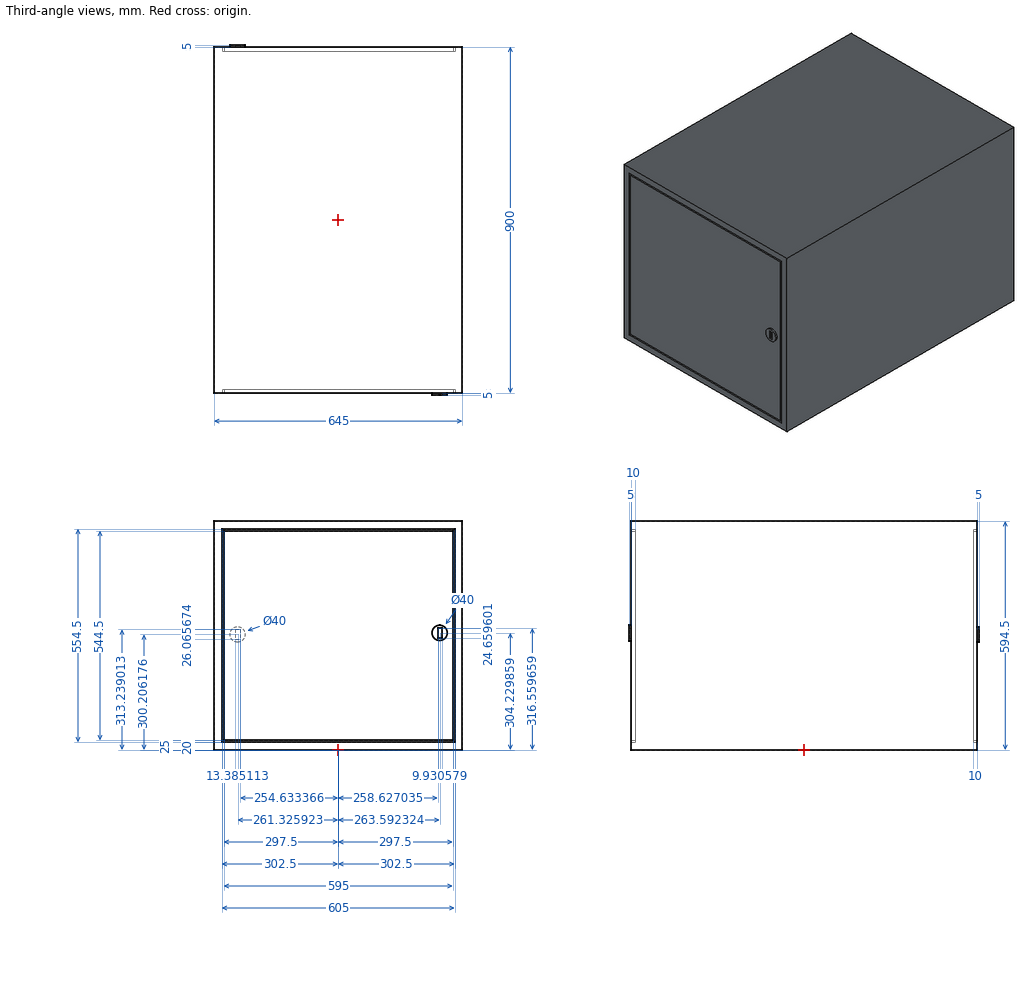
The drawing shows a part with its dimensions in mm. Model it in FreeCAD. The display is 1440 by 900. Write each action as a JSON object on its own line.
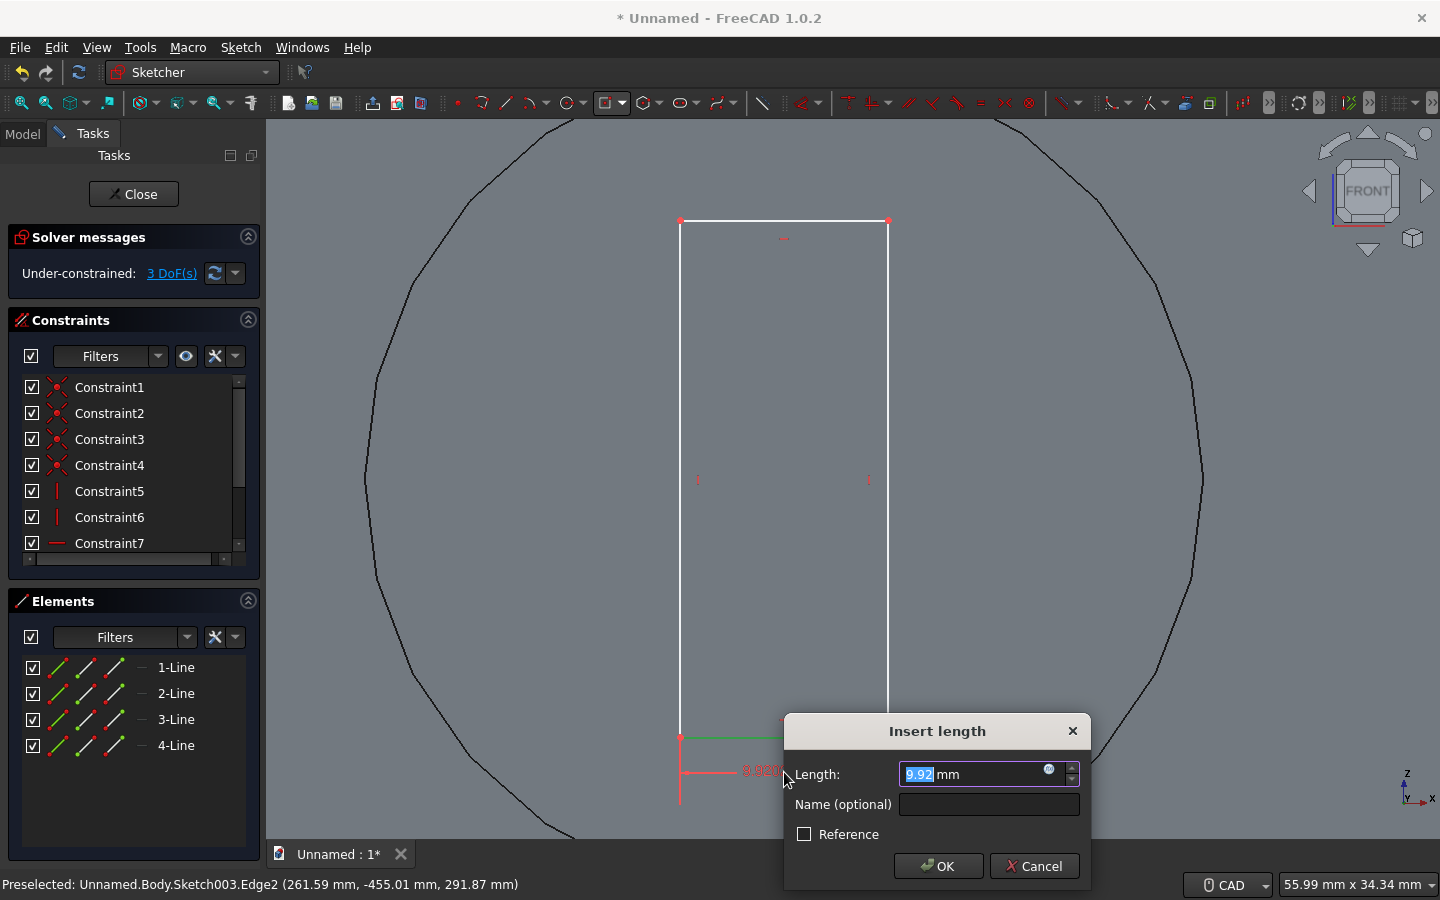
{"action": "type", "text": "9.930579"}
{"action": "key", "text": "Return"}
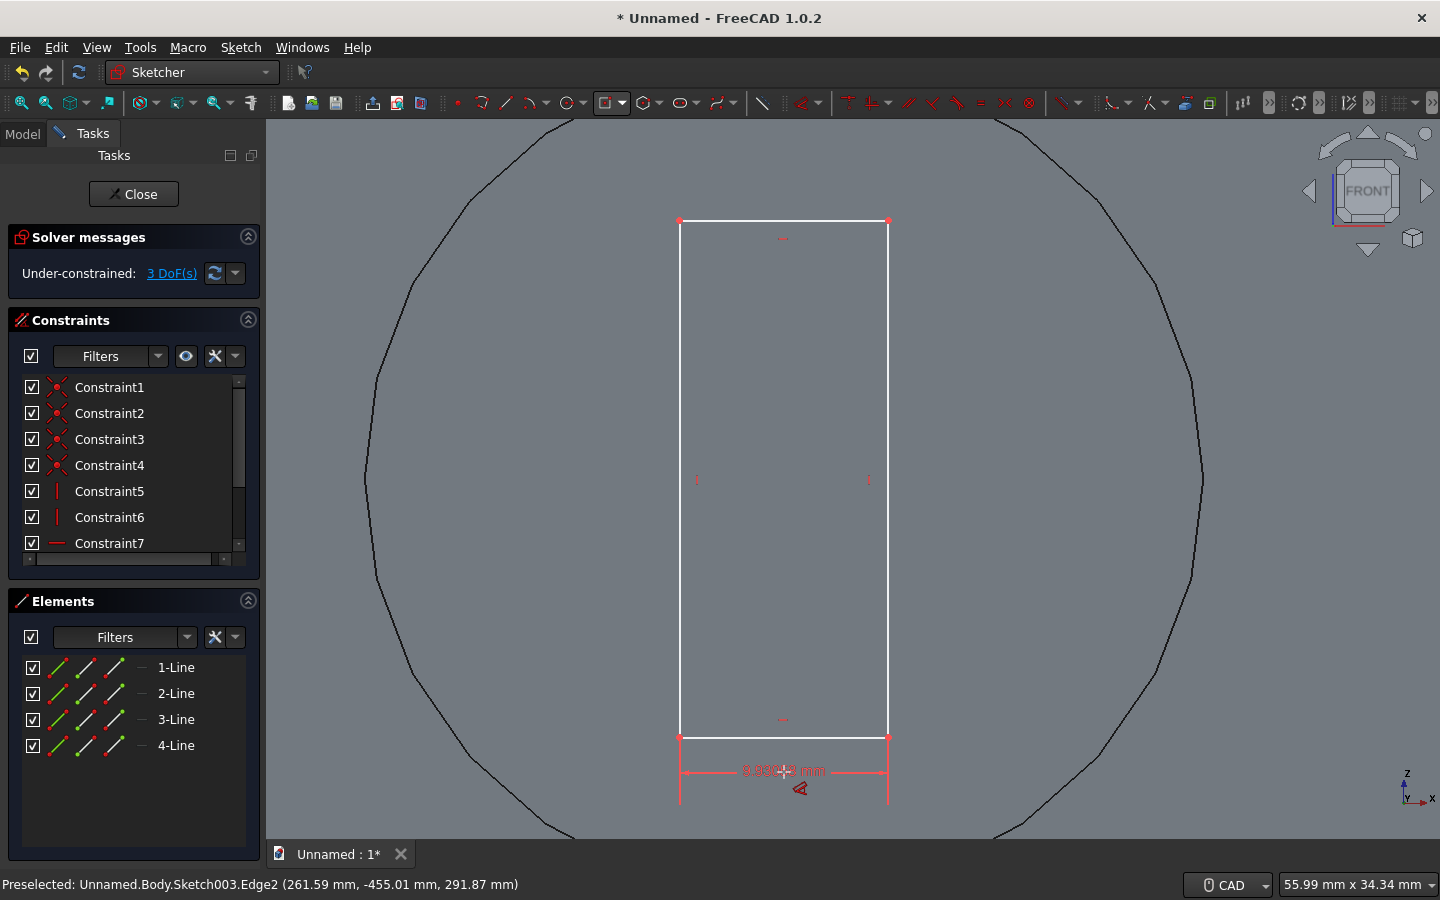
{"action": "left_click", "coordinate": [680, 376]}
{"action": "left_click", "coordinate": [646, 479]}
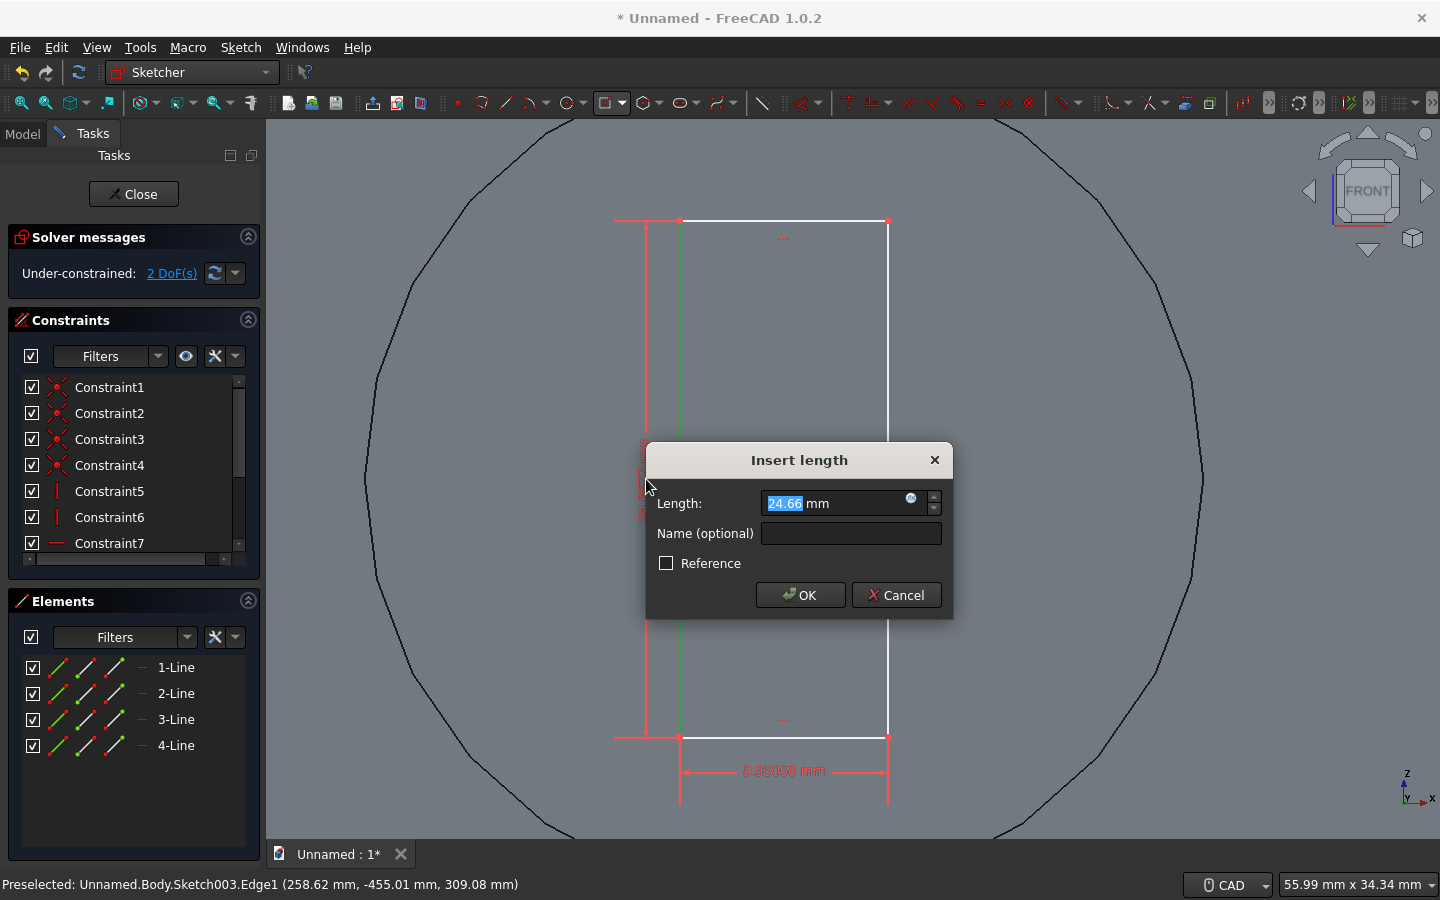
{"action": "type", "text": "24.659601"}
{"action": "key", "text": "Return"}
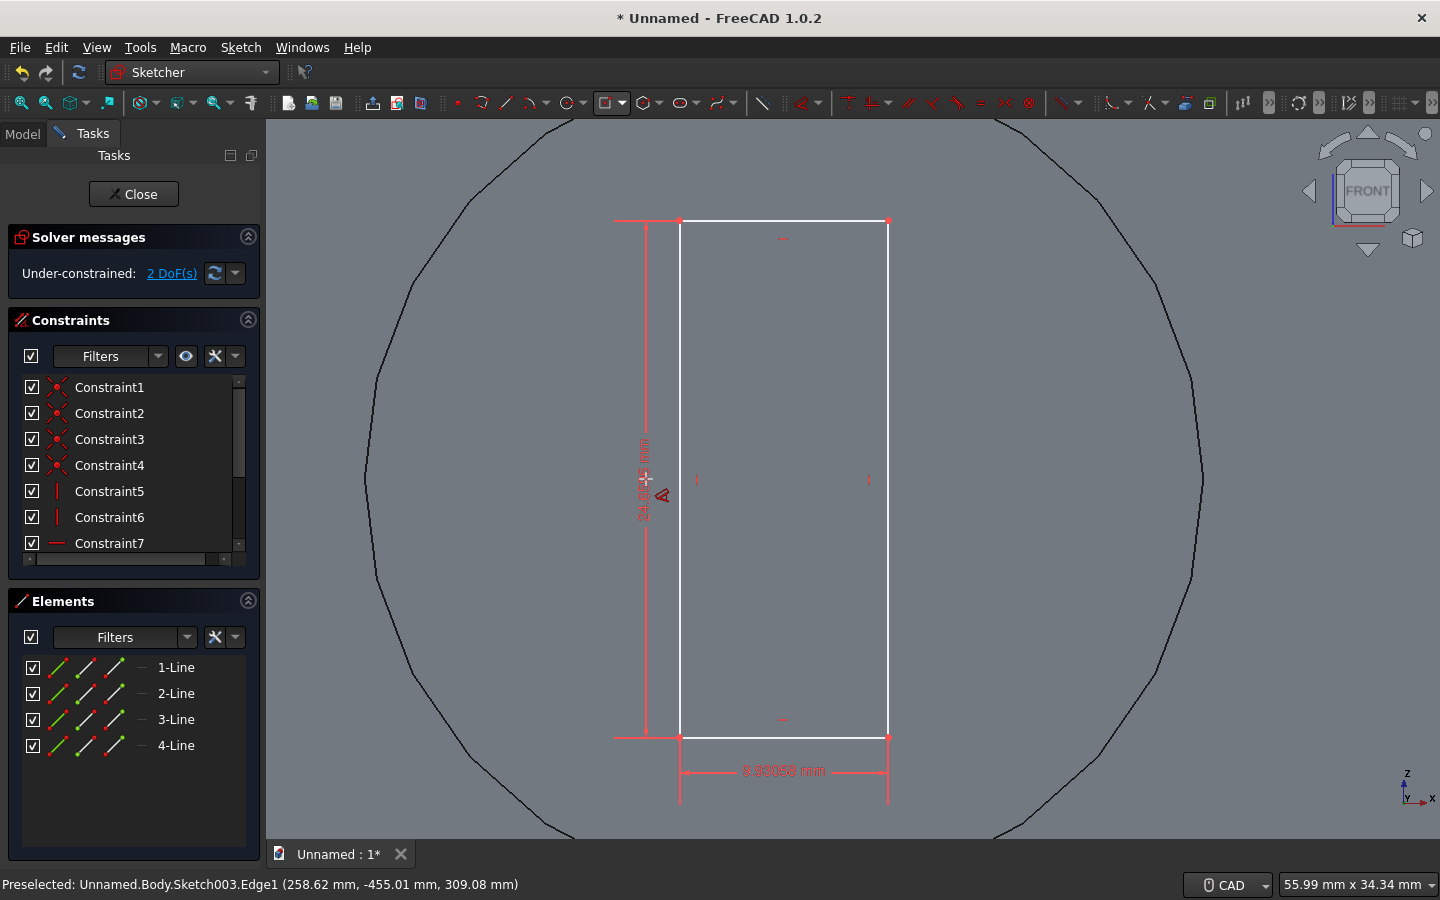
{"action": "left_click", "coordinate": [680, 221]}
{"action": "left_click", "coordinate": [487, 187]}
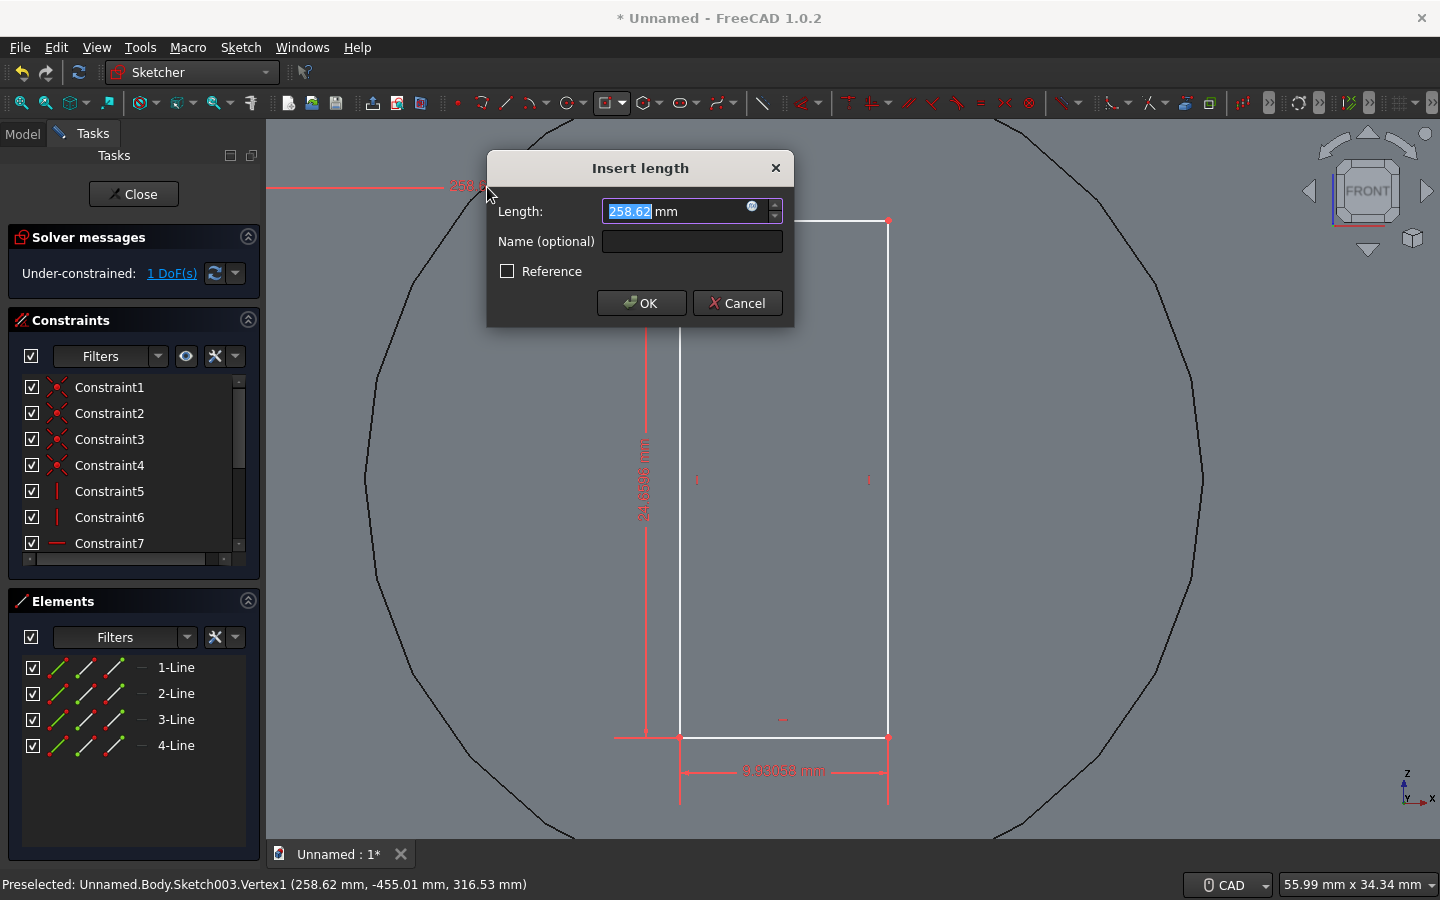
{"action": "type", "text": "258.627035"}
{"action": "key", "text": "Return"}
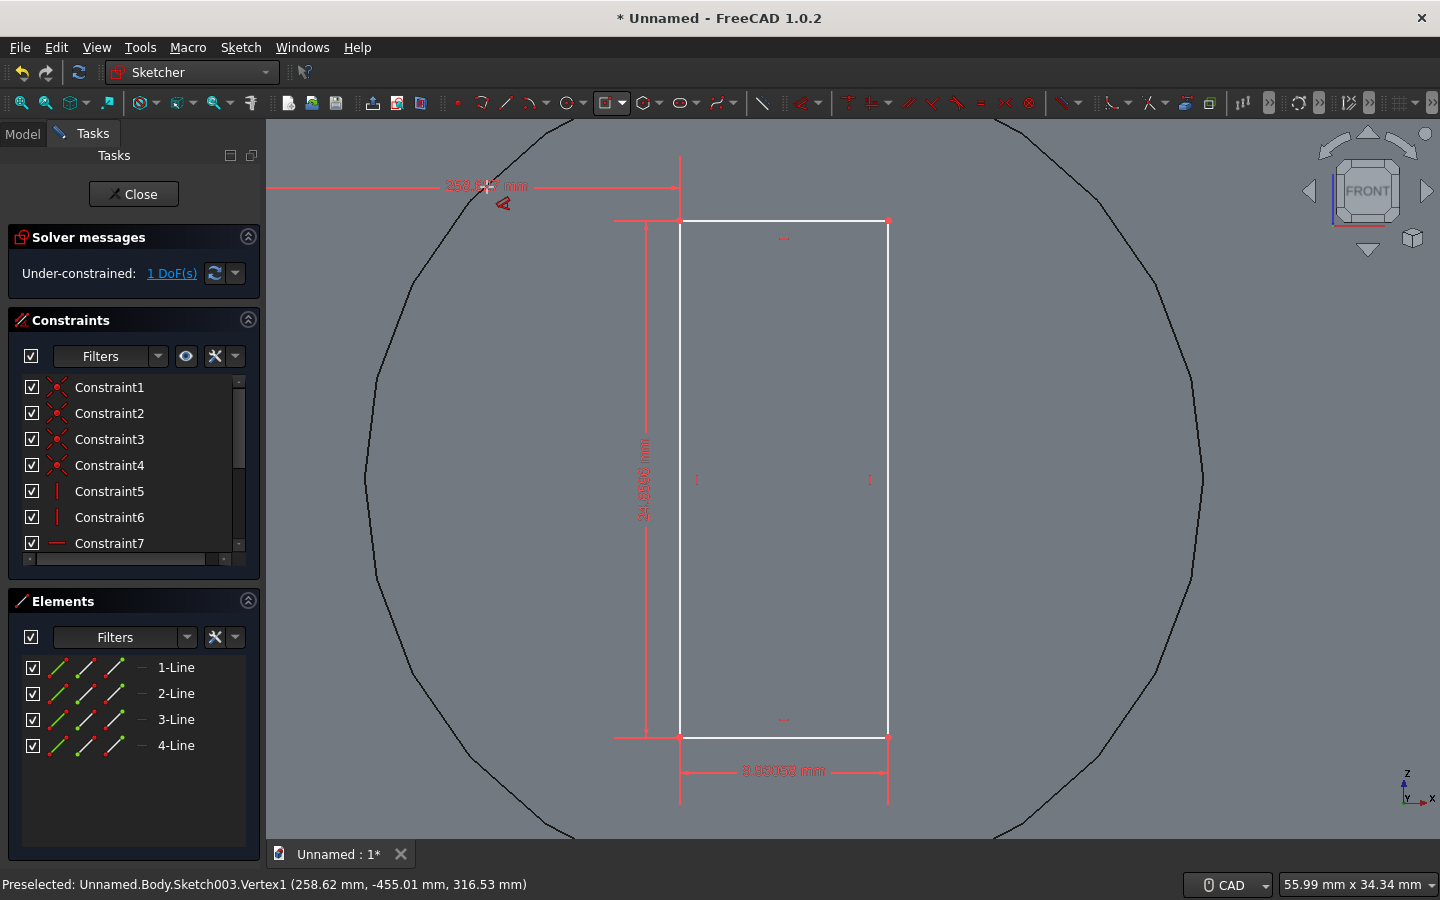
{"action": "left_click", "coordinate": [680, 221]}
{"action": "left_click", "coordinate": [714, 516]}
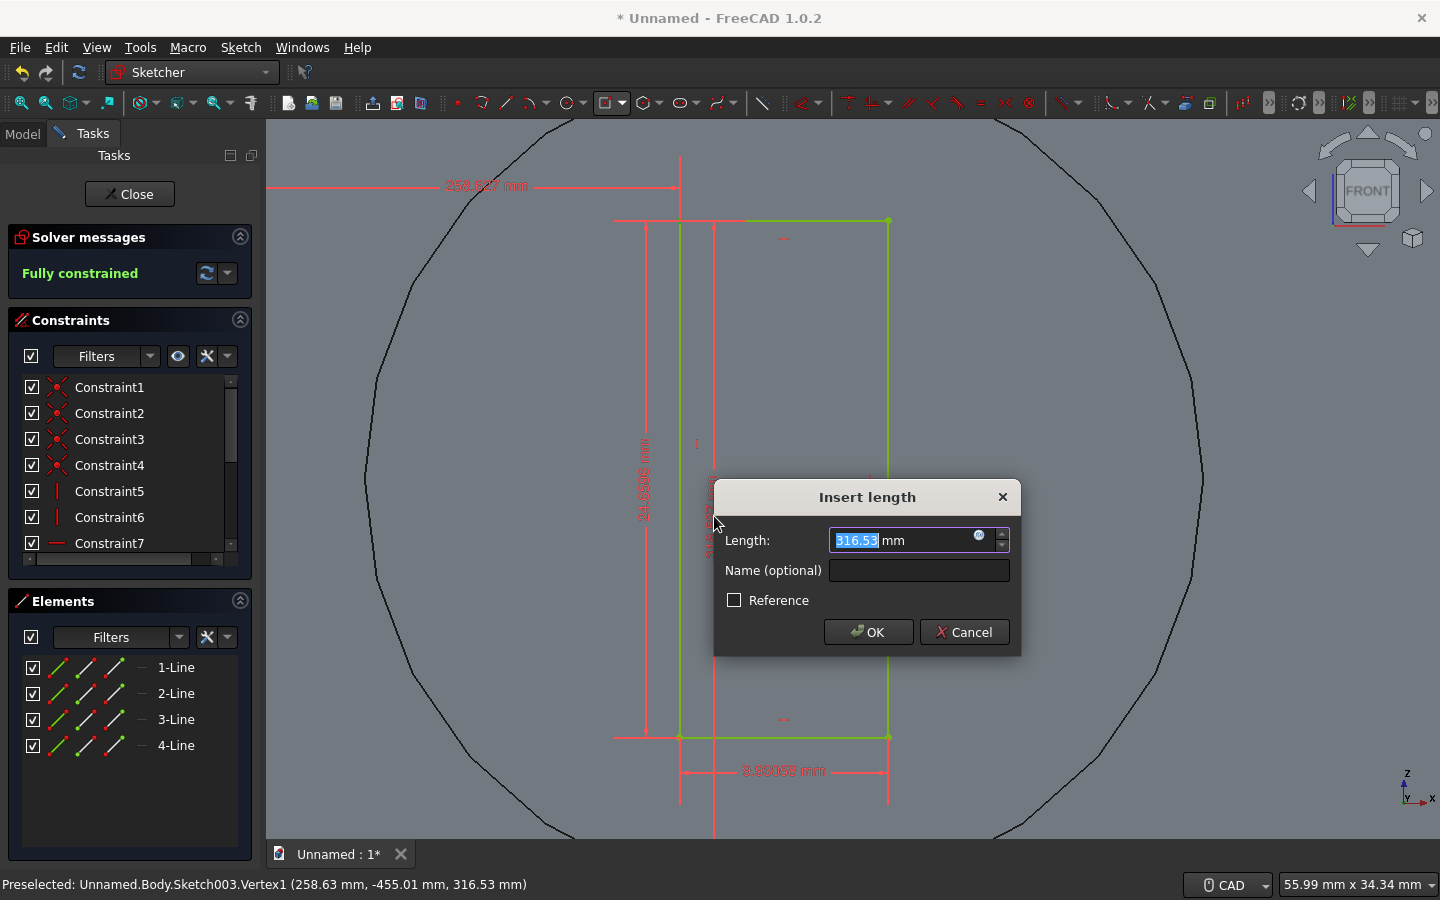
{"action": "type", "text": "316.559659"}
{"action": "key", "text": "Return"}
{"action": "key", "text": "Escape"}